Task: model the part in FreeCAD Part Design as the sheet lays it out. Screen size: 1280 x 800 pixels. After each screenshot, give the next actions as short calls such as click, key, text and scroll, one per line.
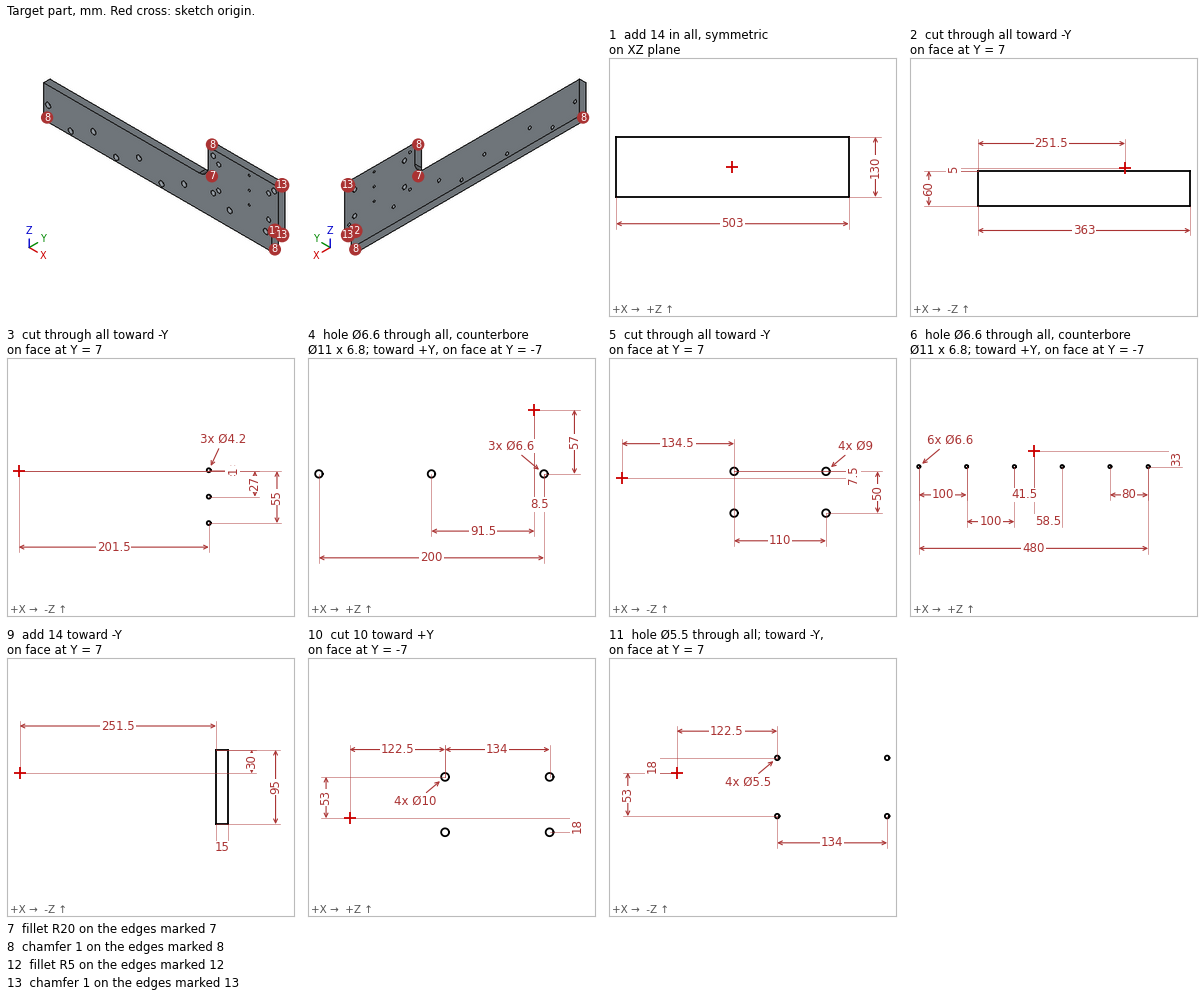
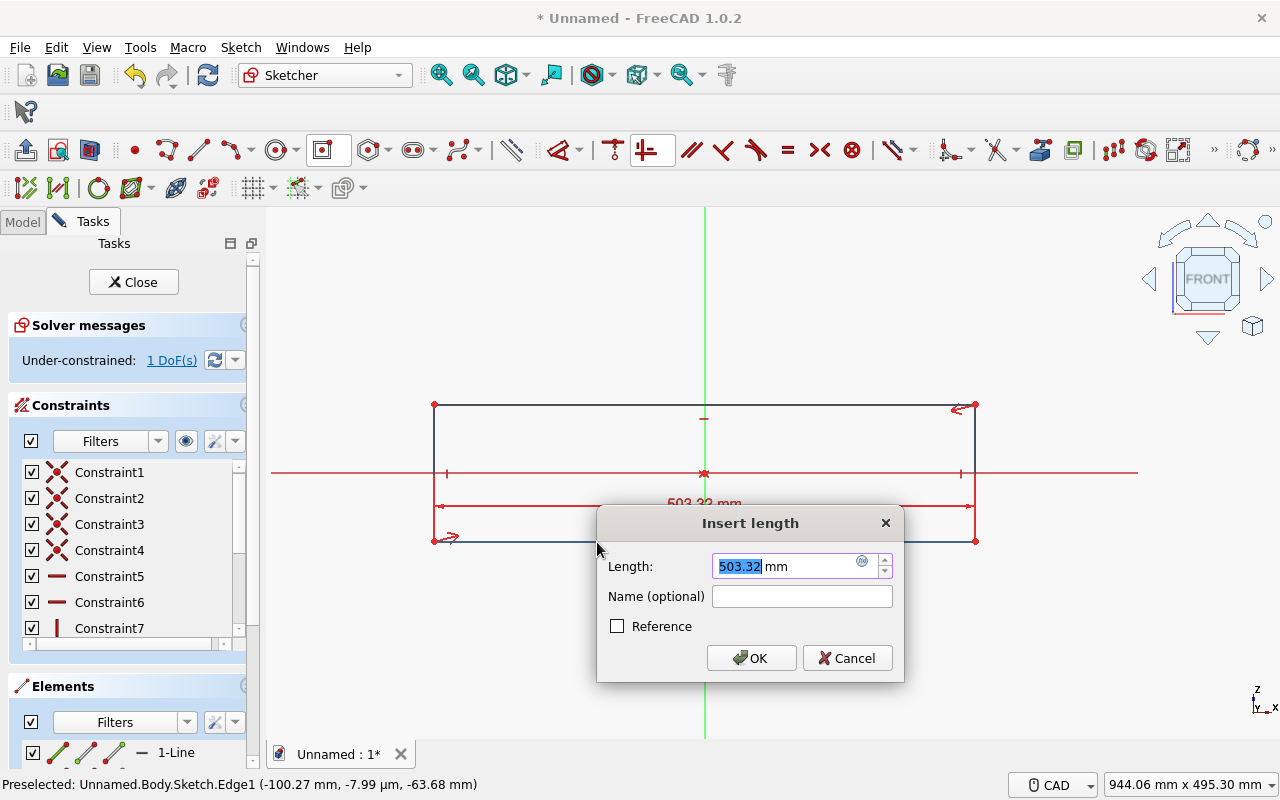
text(503)
key(Return)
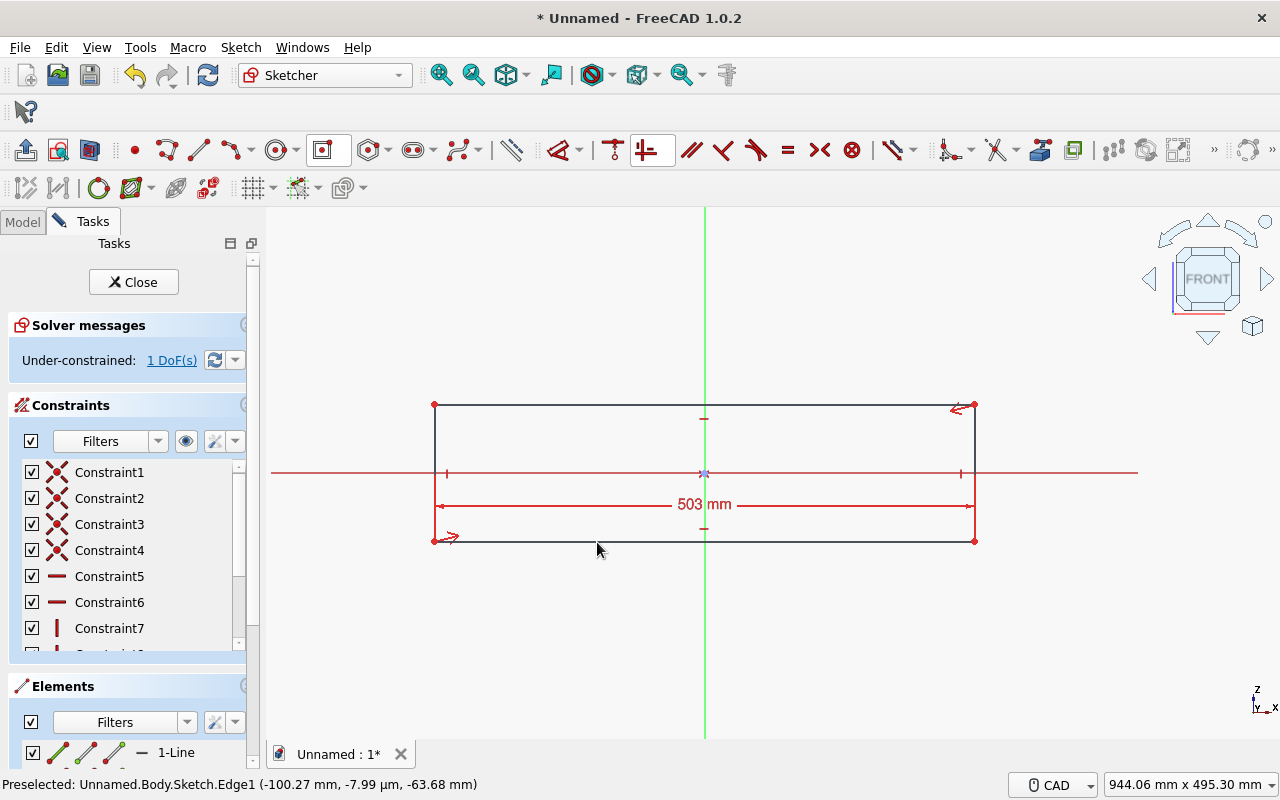
click(975, 501)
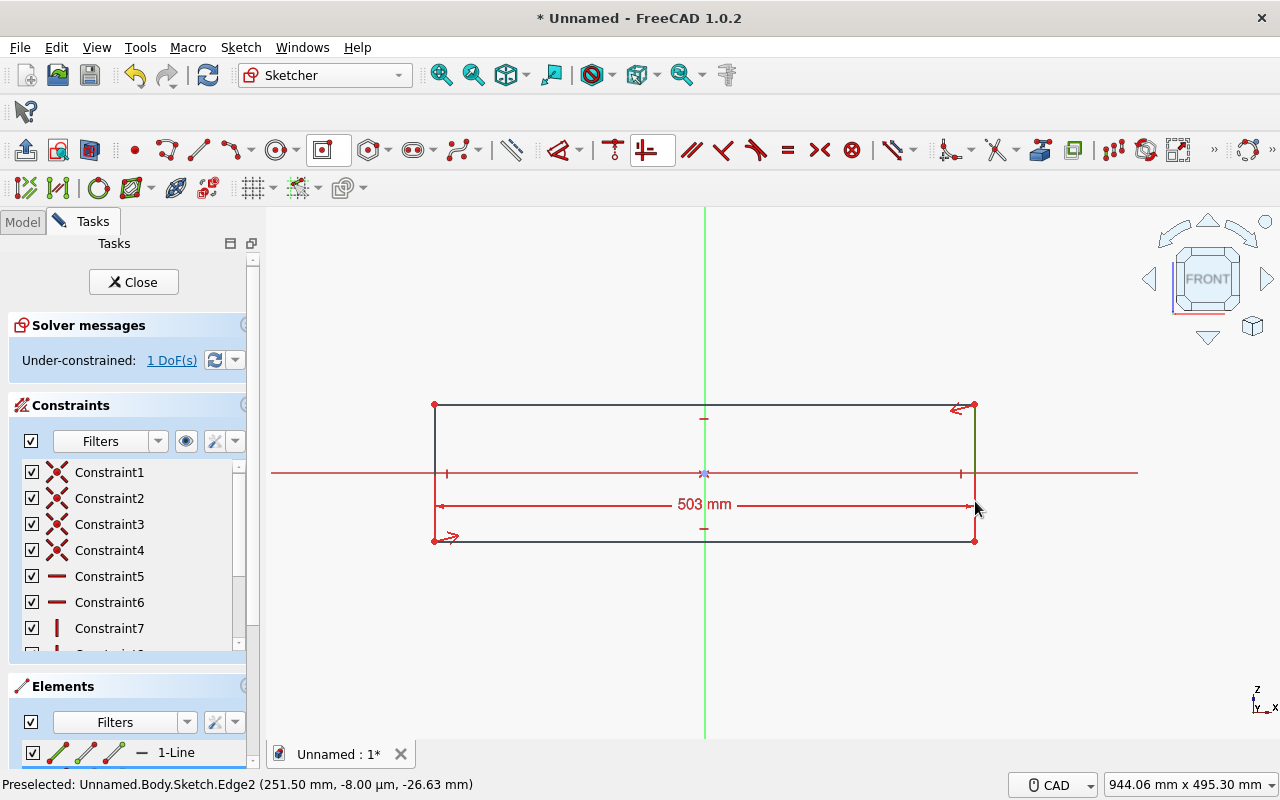
key(i)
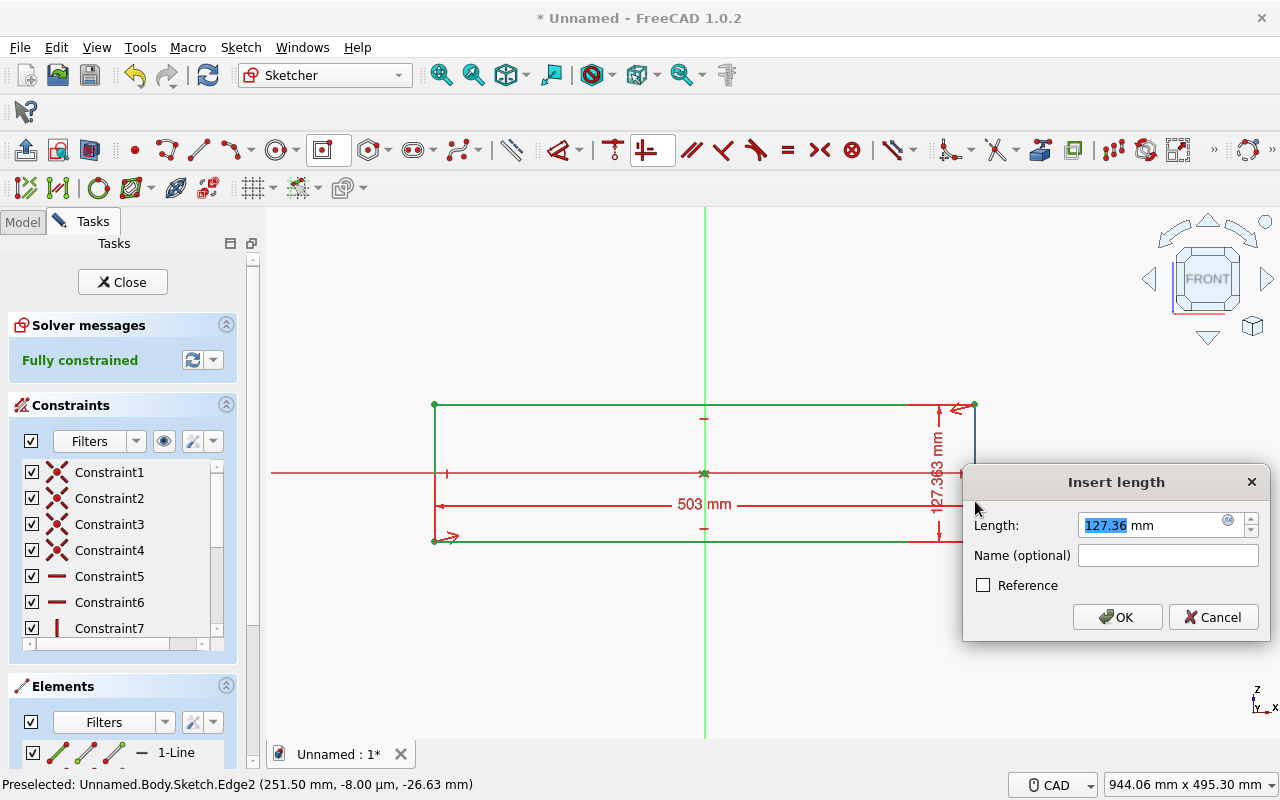
text(130)
key(Return)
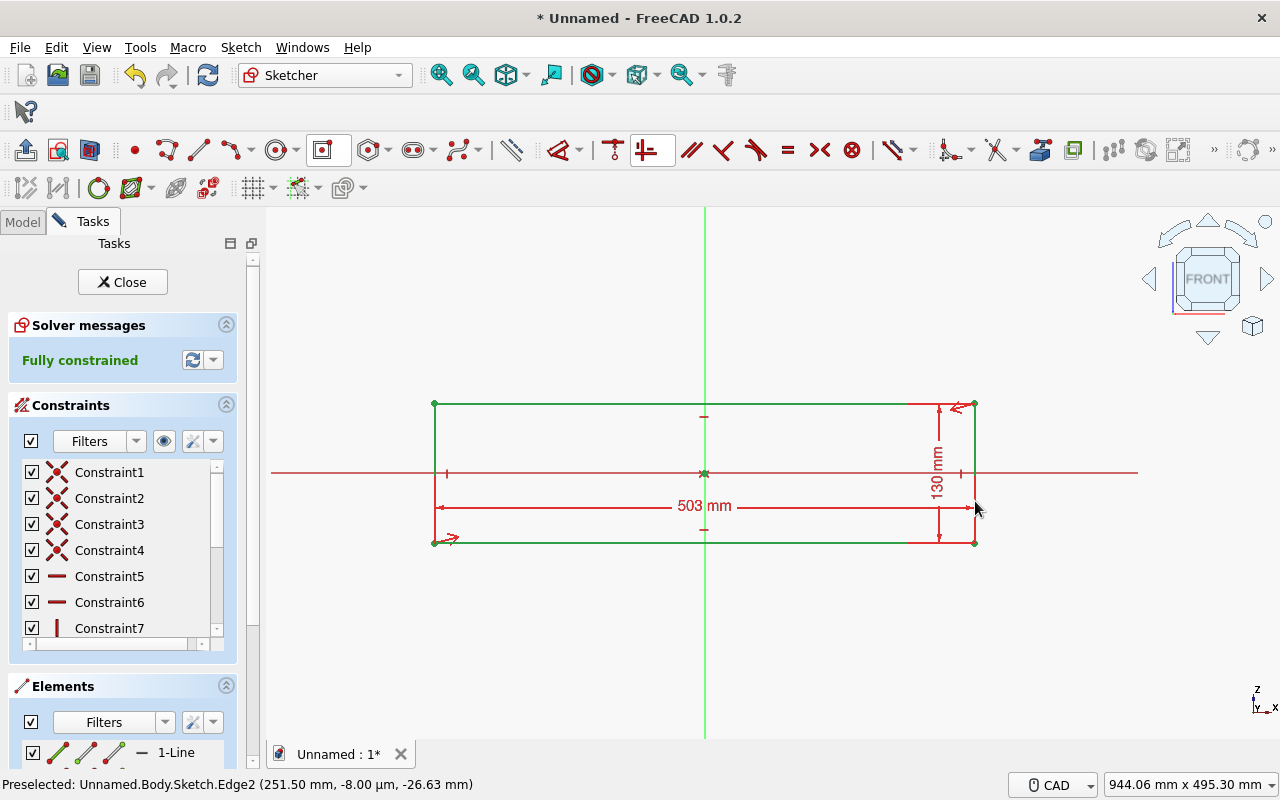
click(123, 282)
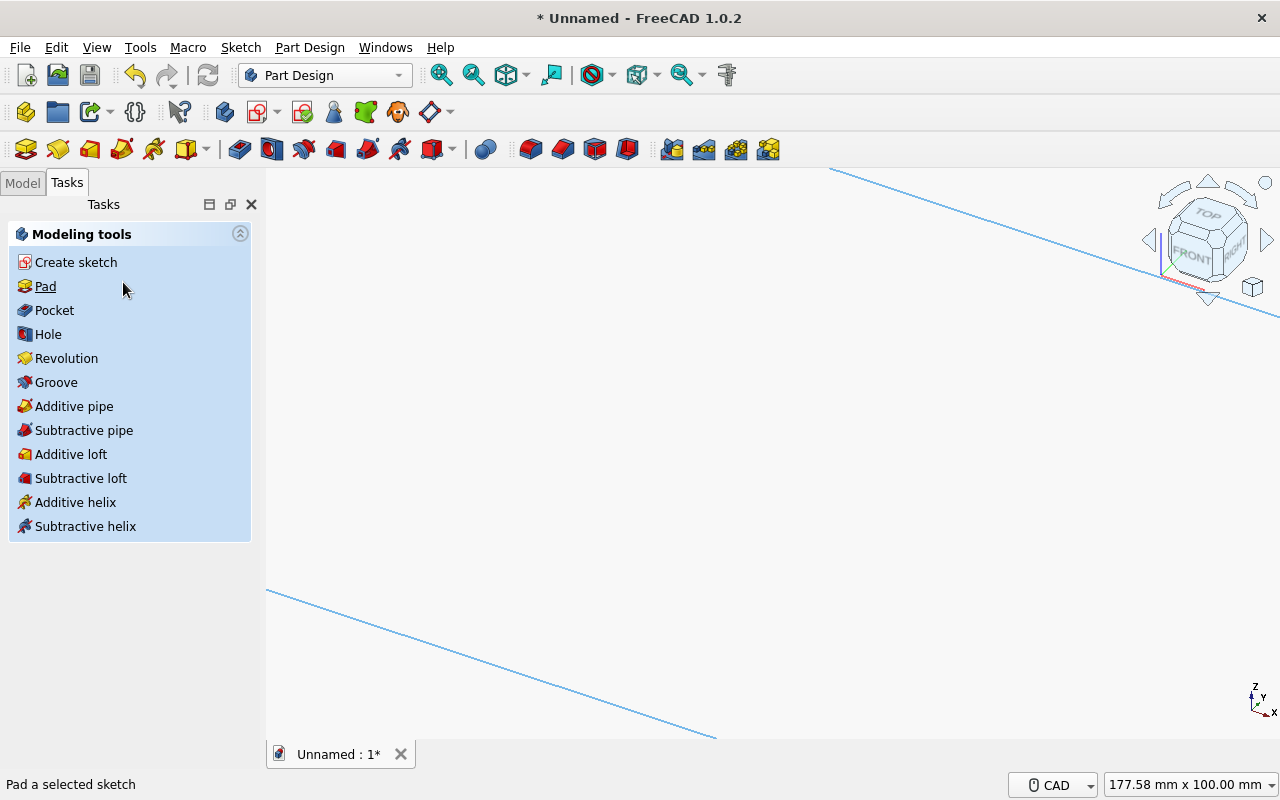
click(26, 150)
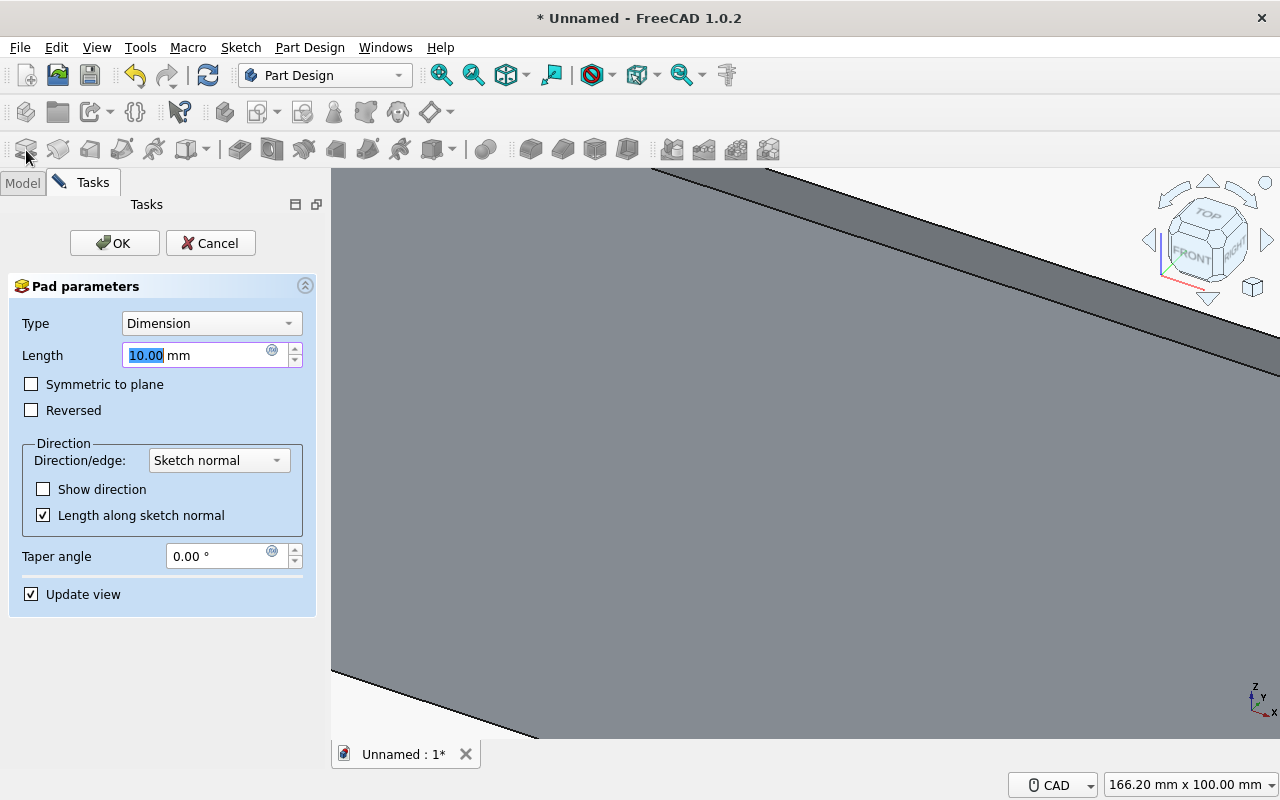
text(14)
key(Tab)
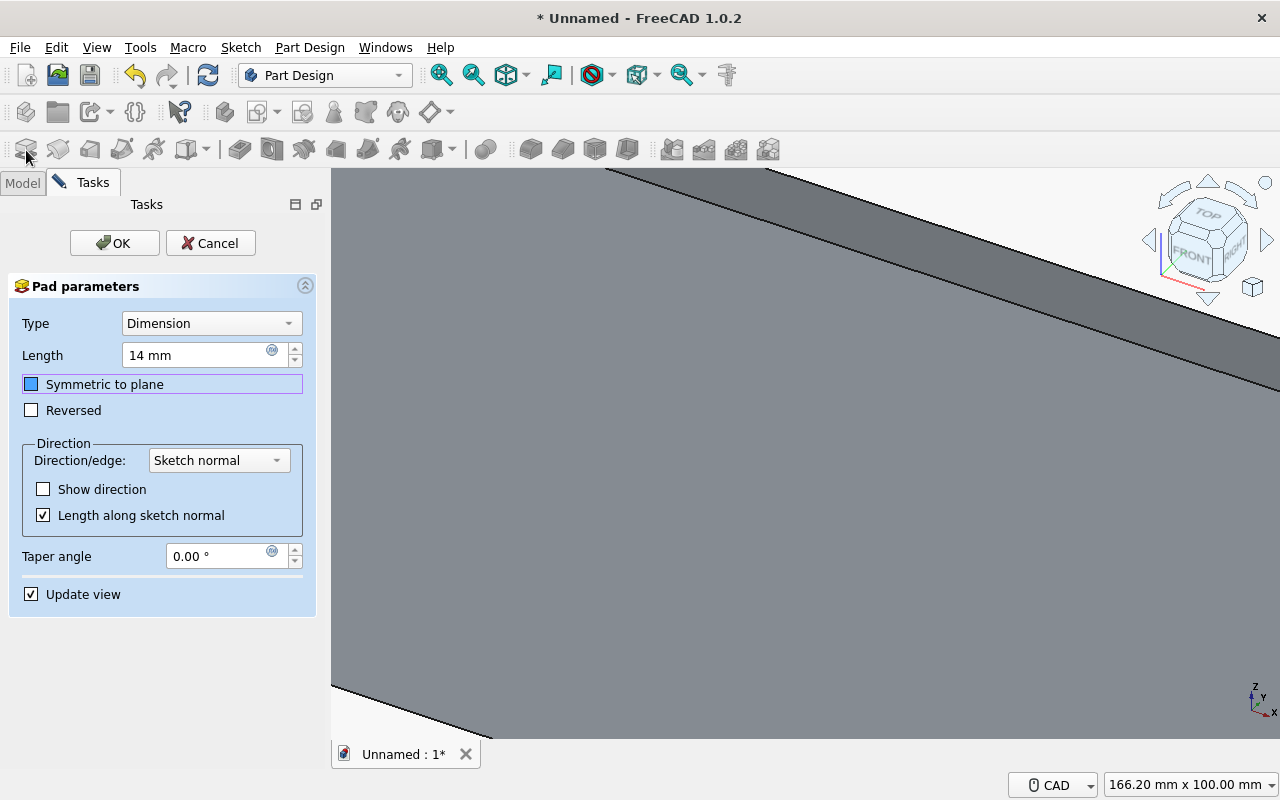
click(30, 384)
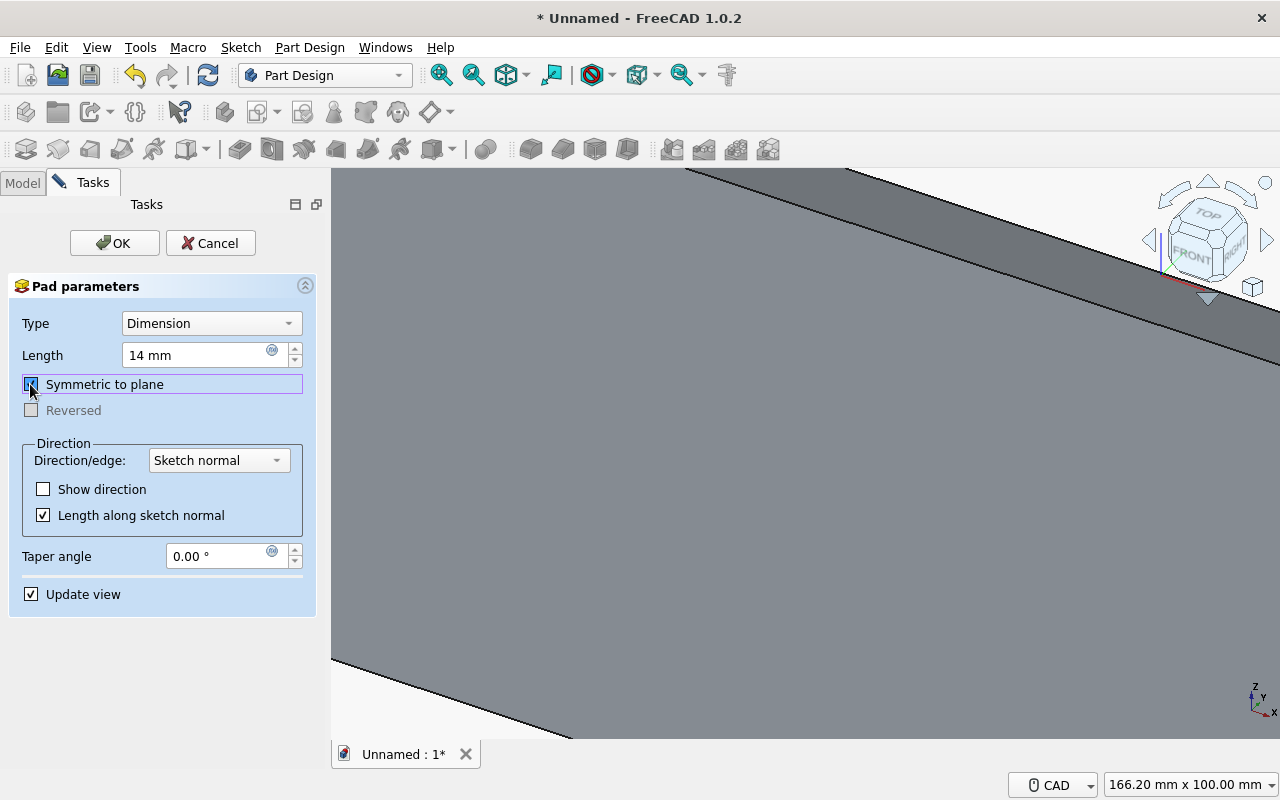
click(115, 243)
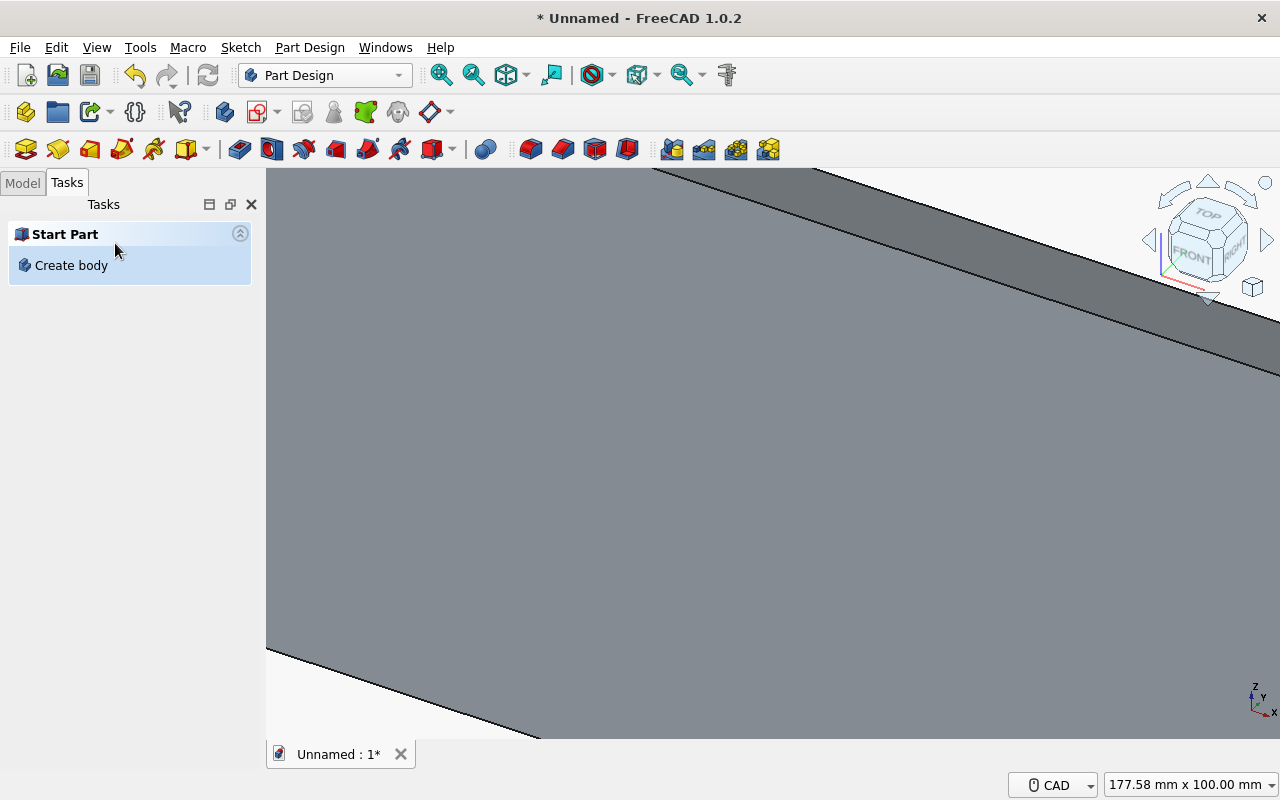
key(v)
key(f)